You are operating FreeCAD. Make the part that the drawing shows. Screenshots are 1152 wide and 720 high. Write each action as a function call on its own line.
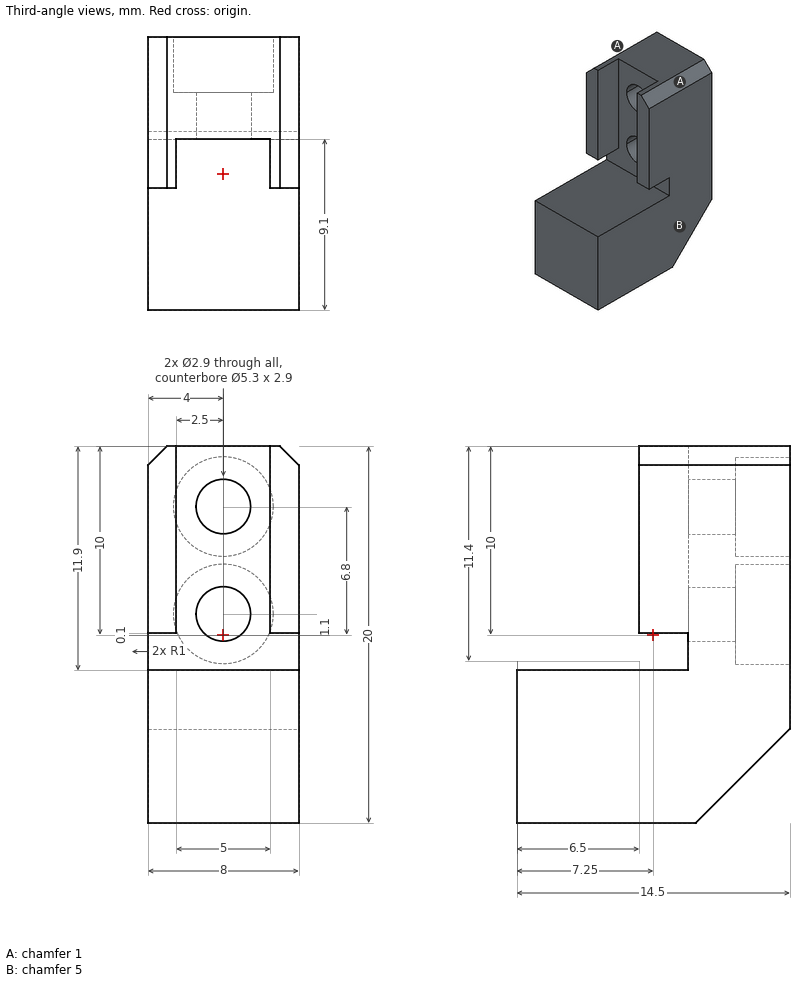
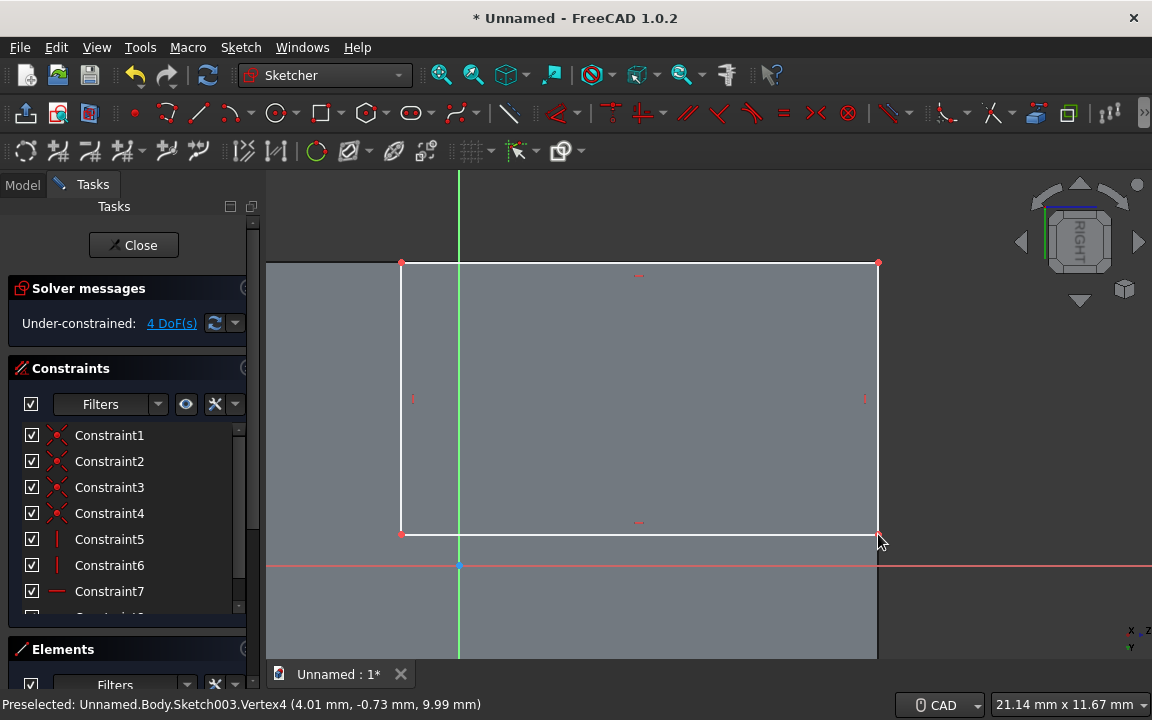
key(d)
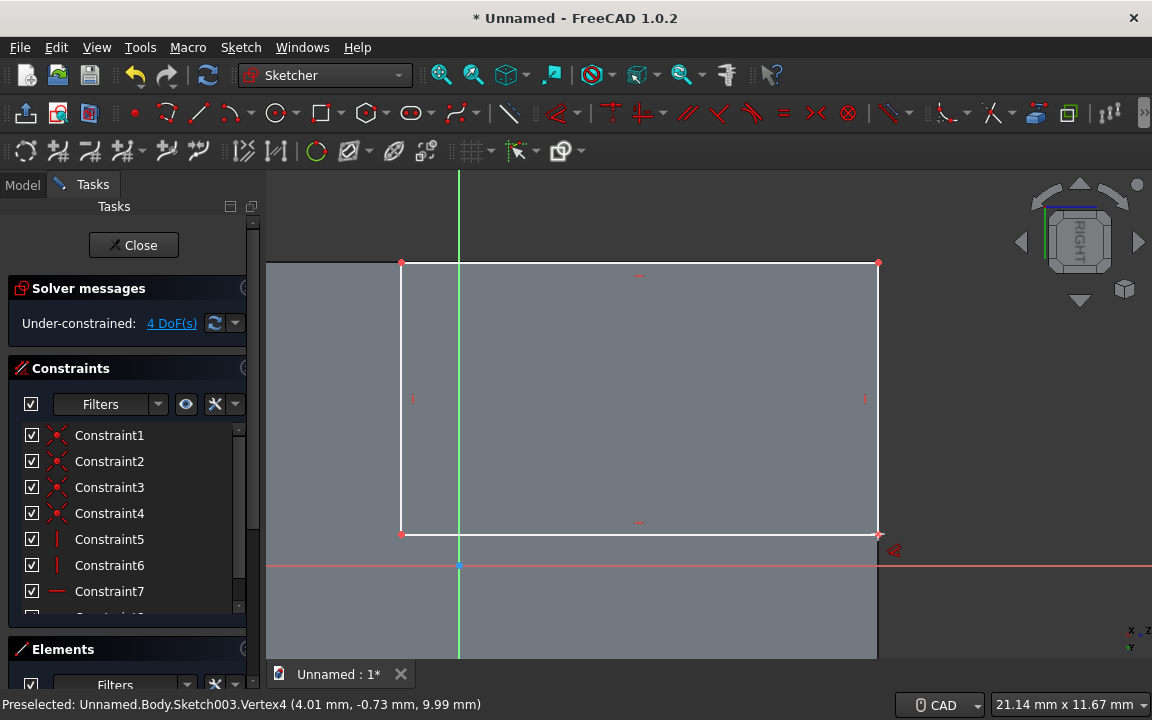
click(401, 345)
click(367, 399)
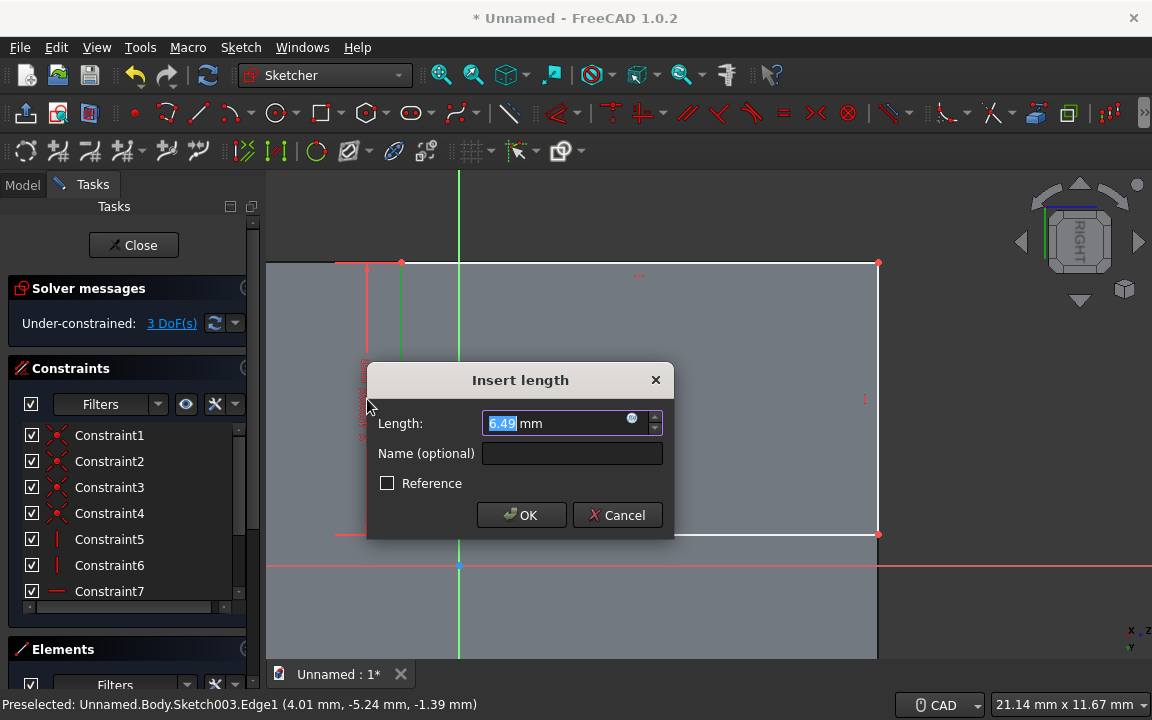
text(6.5)
key(Return)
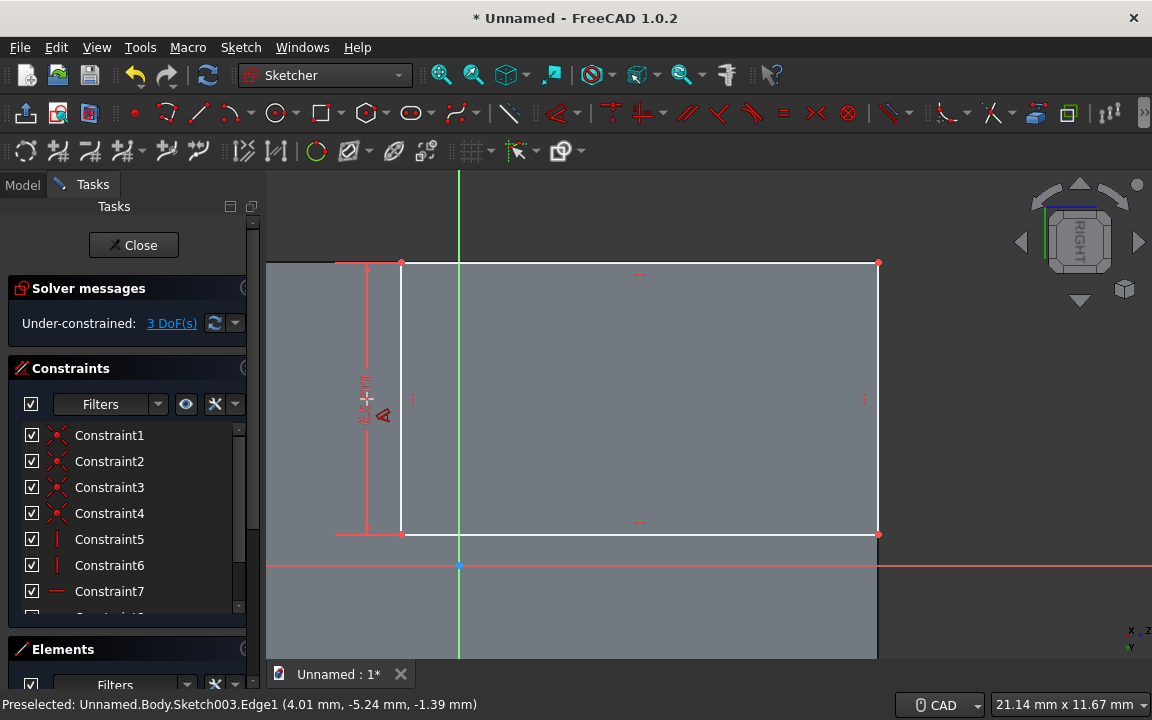
click(878, 535)
click(669, 600)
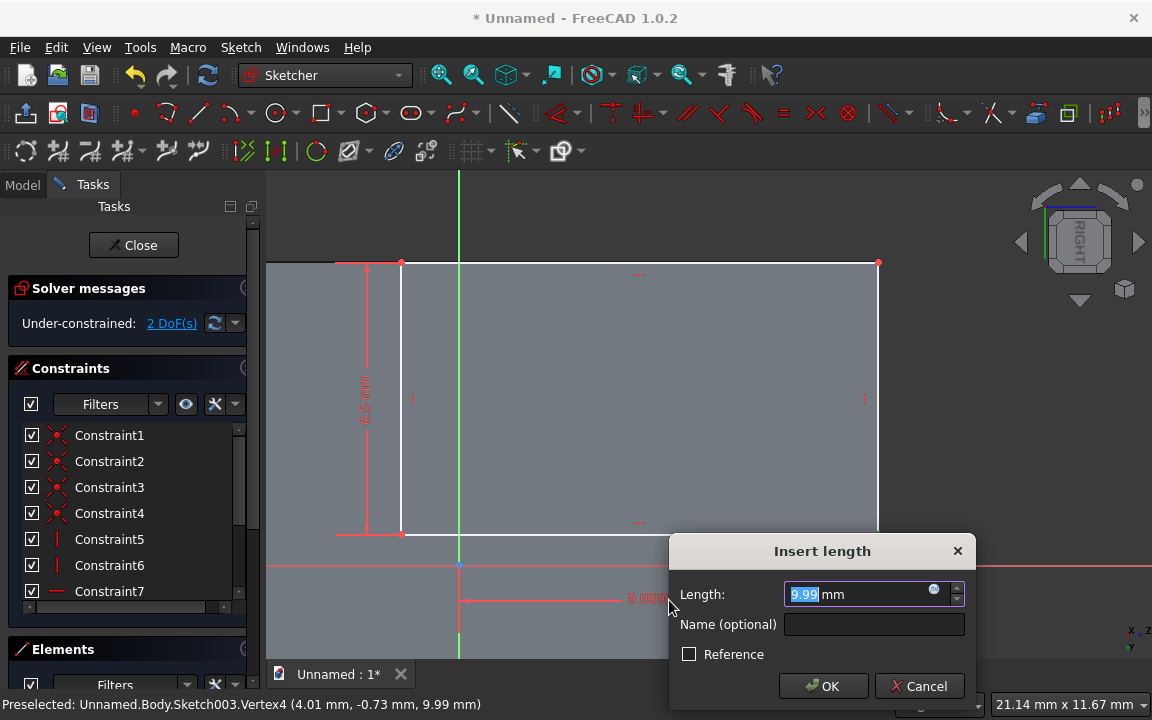
text(10)
key(Return)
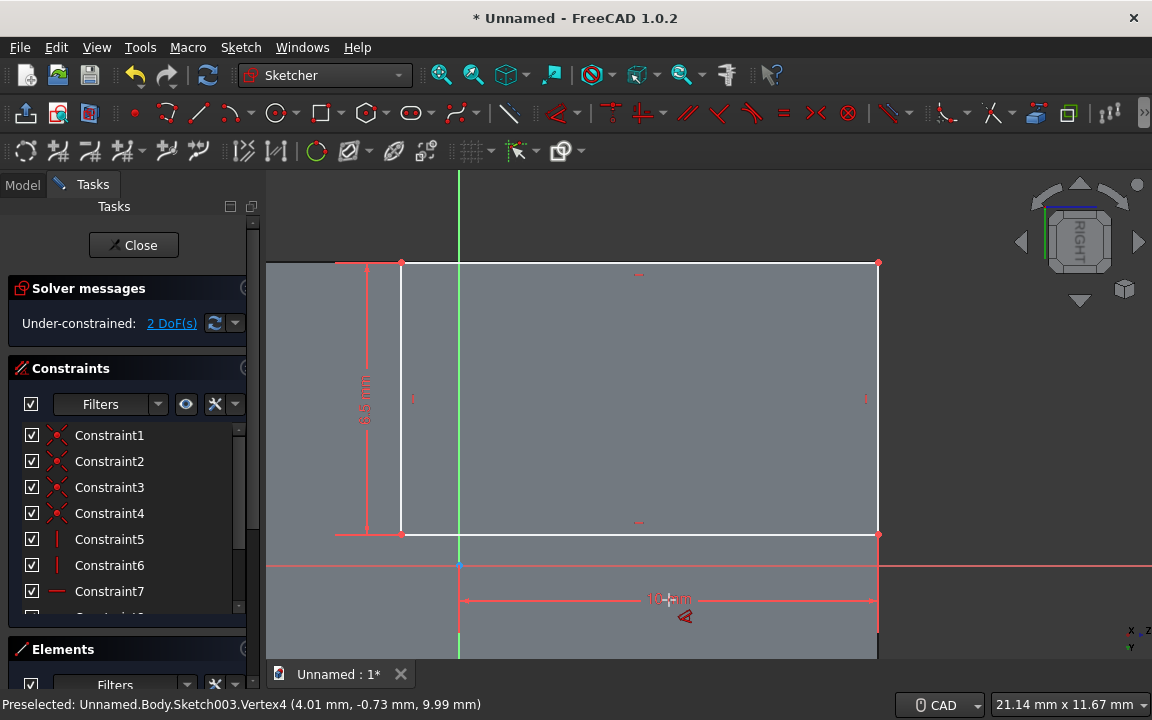
click(544, 535)
click(640, 501)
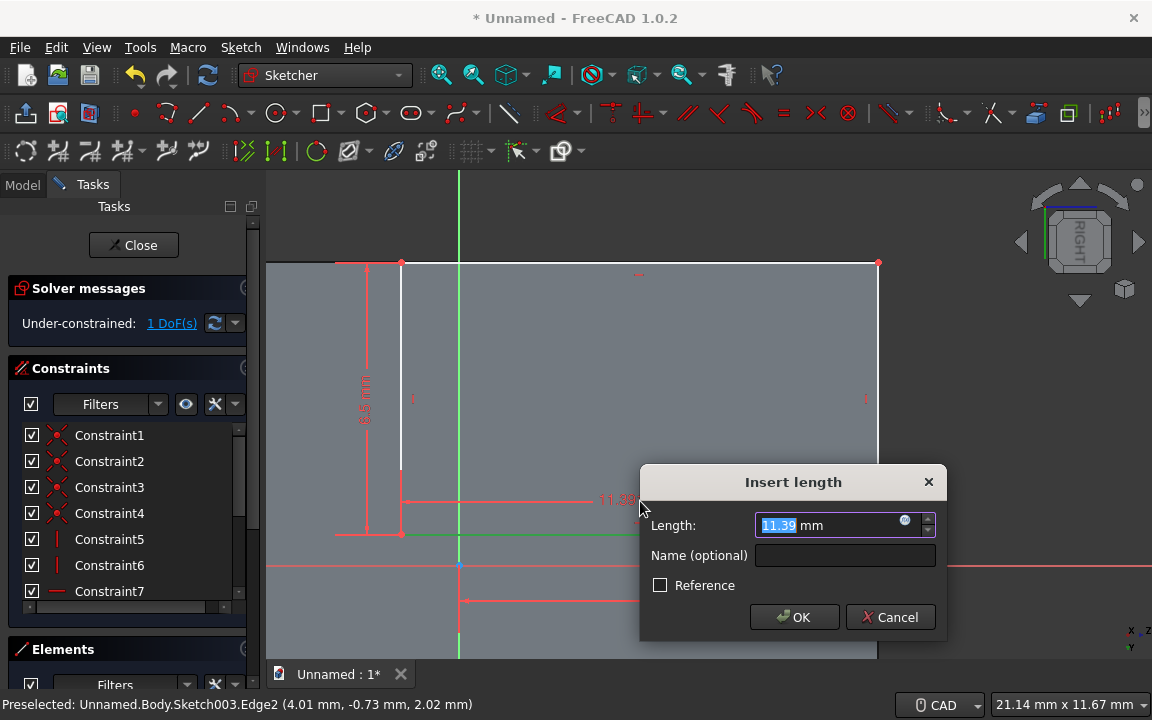
text(11.4)
key(Return)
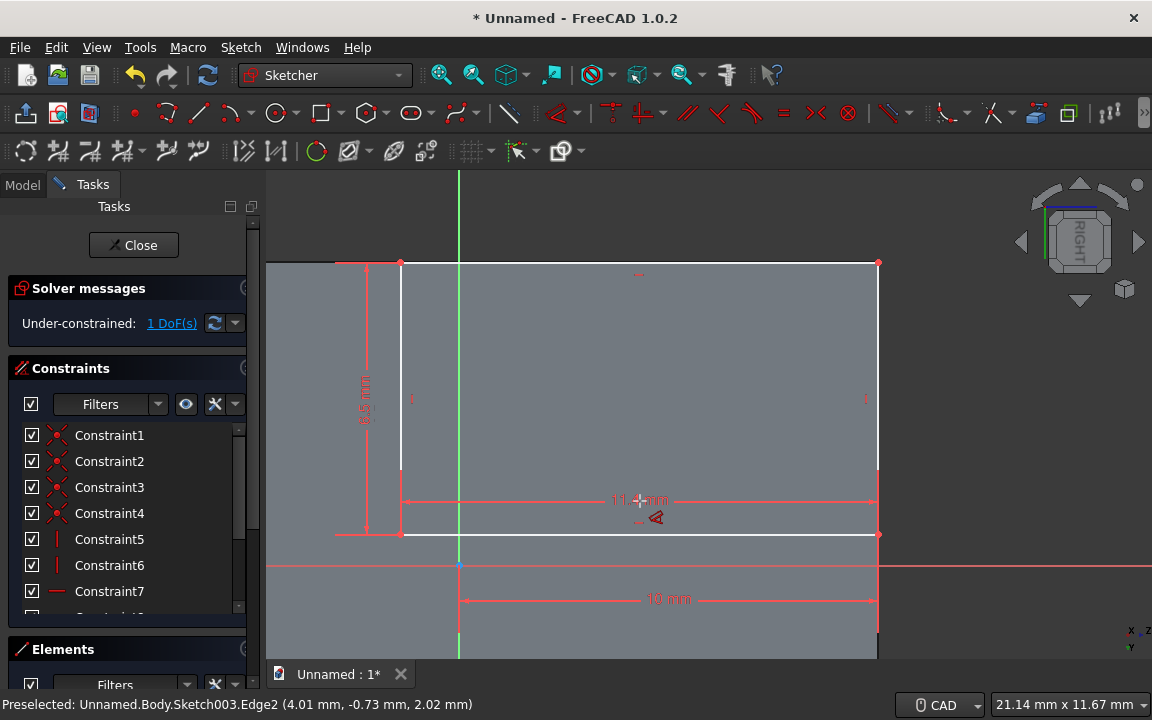
click(401, 263)
click(367, 344)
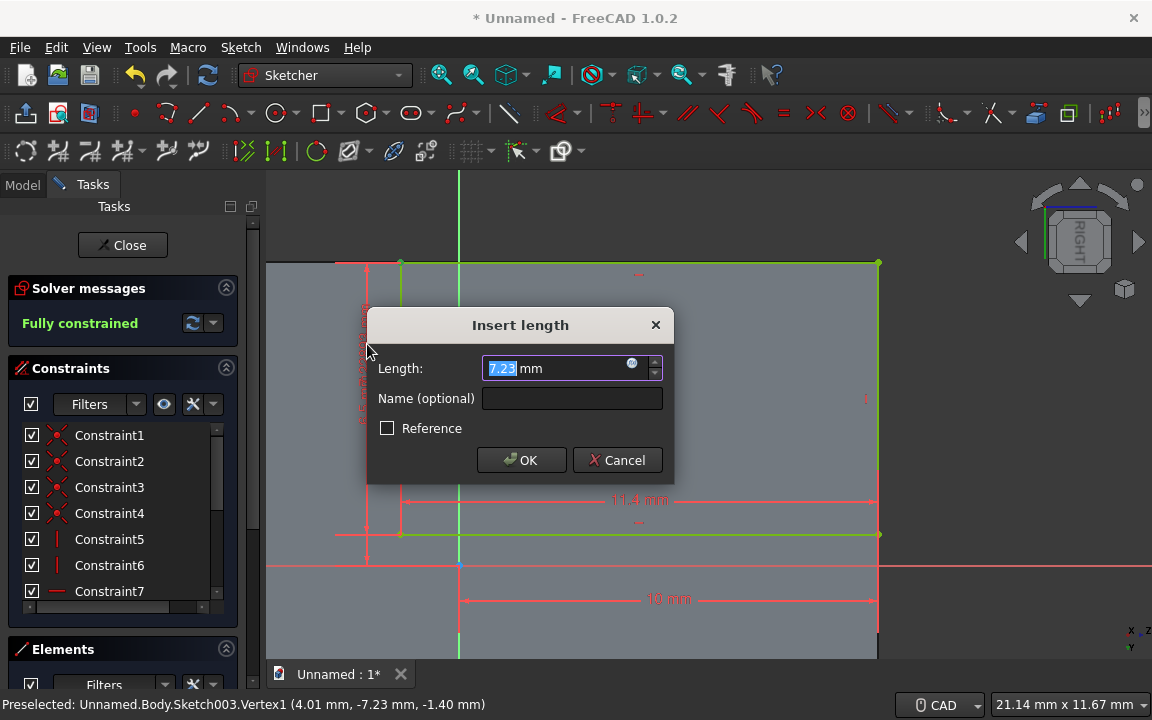
text(7.25)
key(Return)
key(Escape)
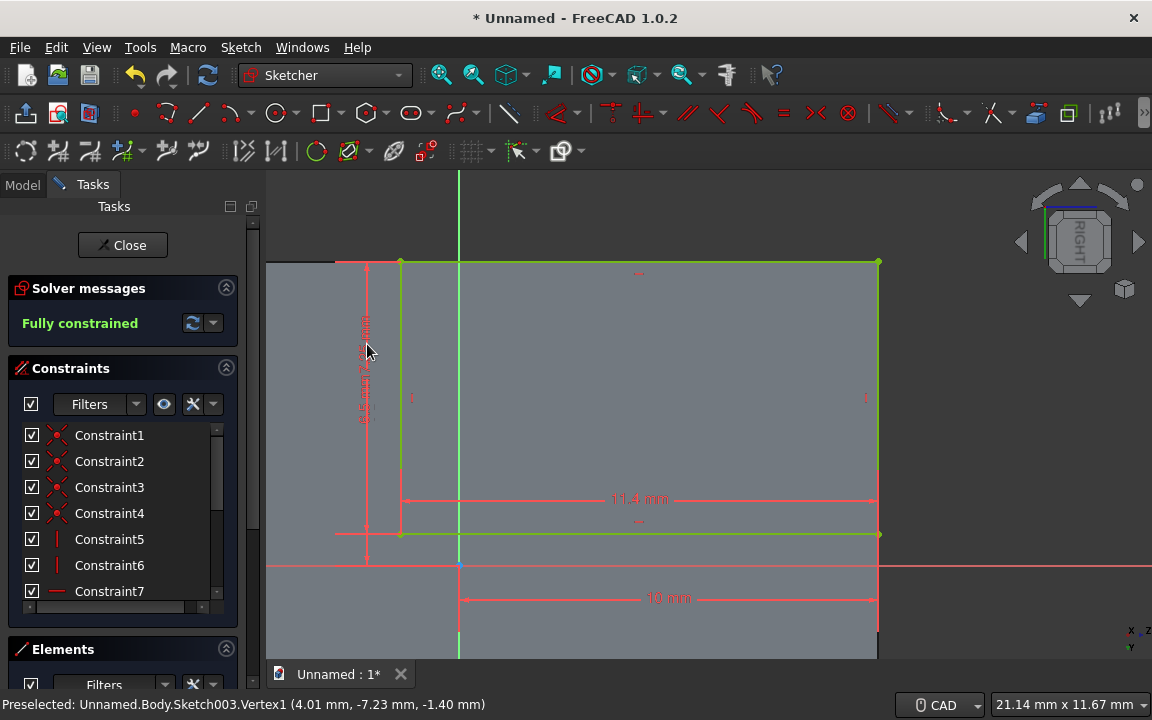
click(123, 245)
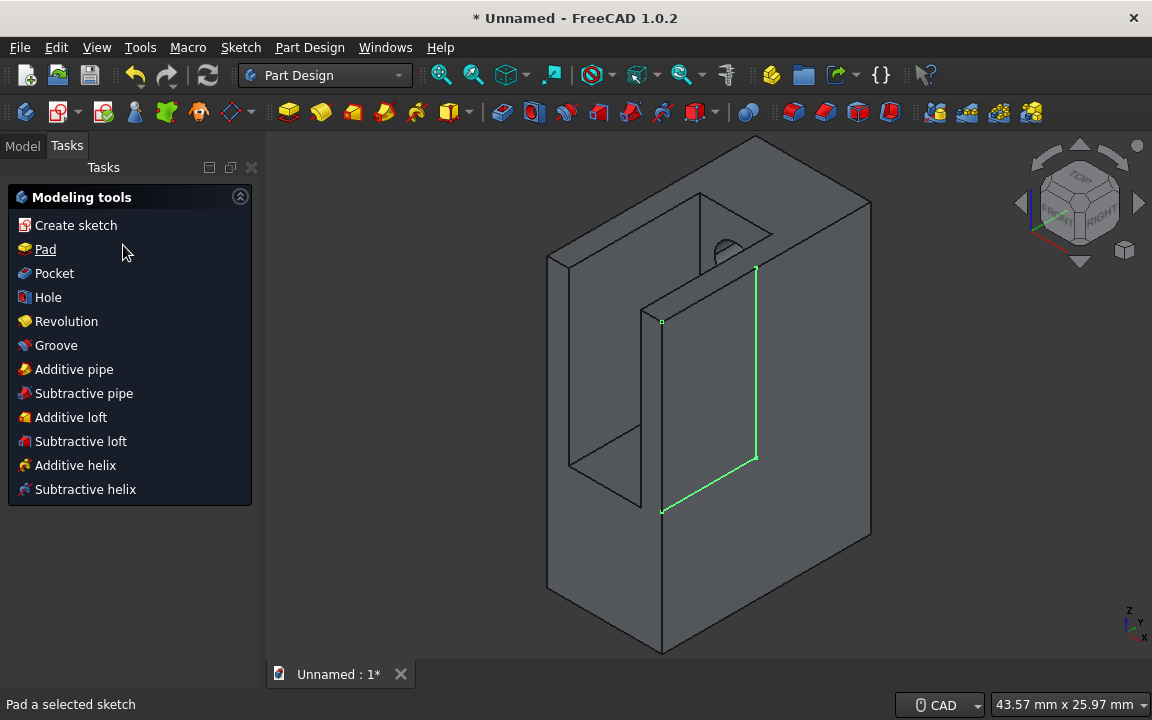
click(504, 112)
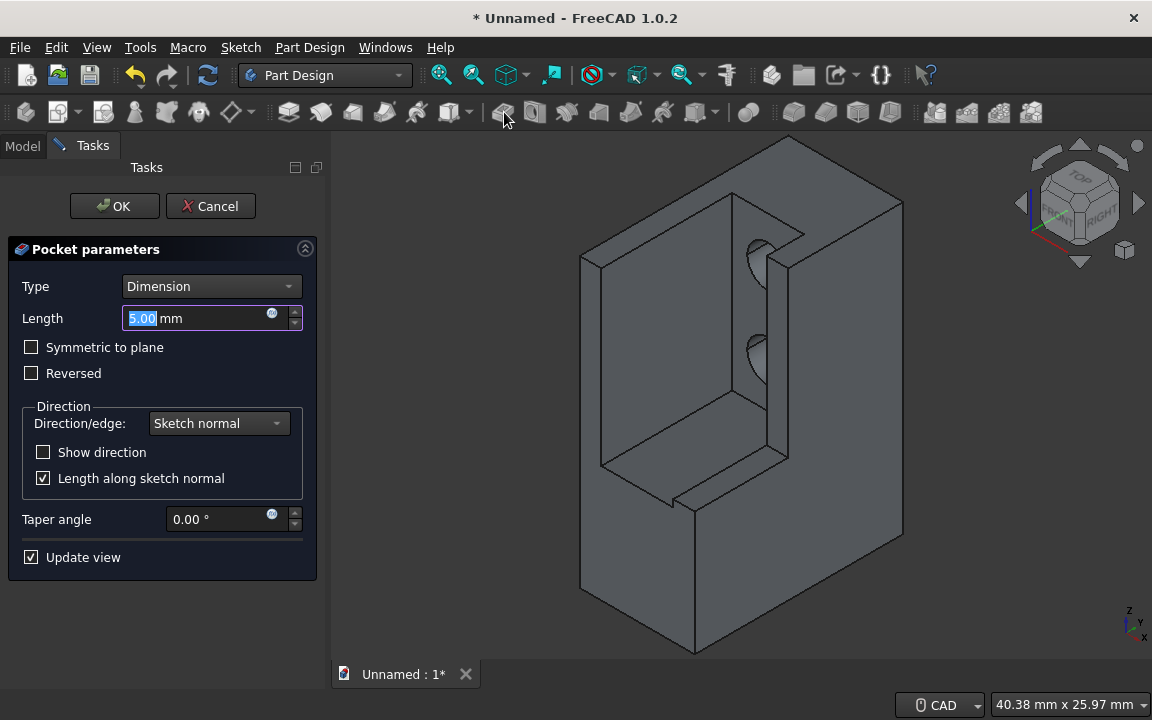
click(212, 286)